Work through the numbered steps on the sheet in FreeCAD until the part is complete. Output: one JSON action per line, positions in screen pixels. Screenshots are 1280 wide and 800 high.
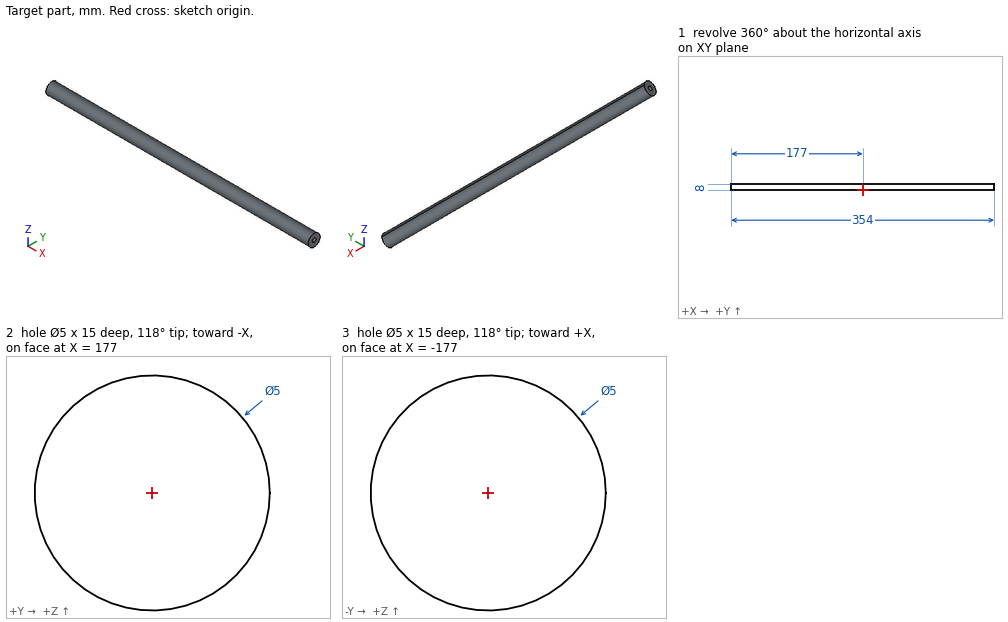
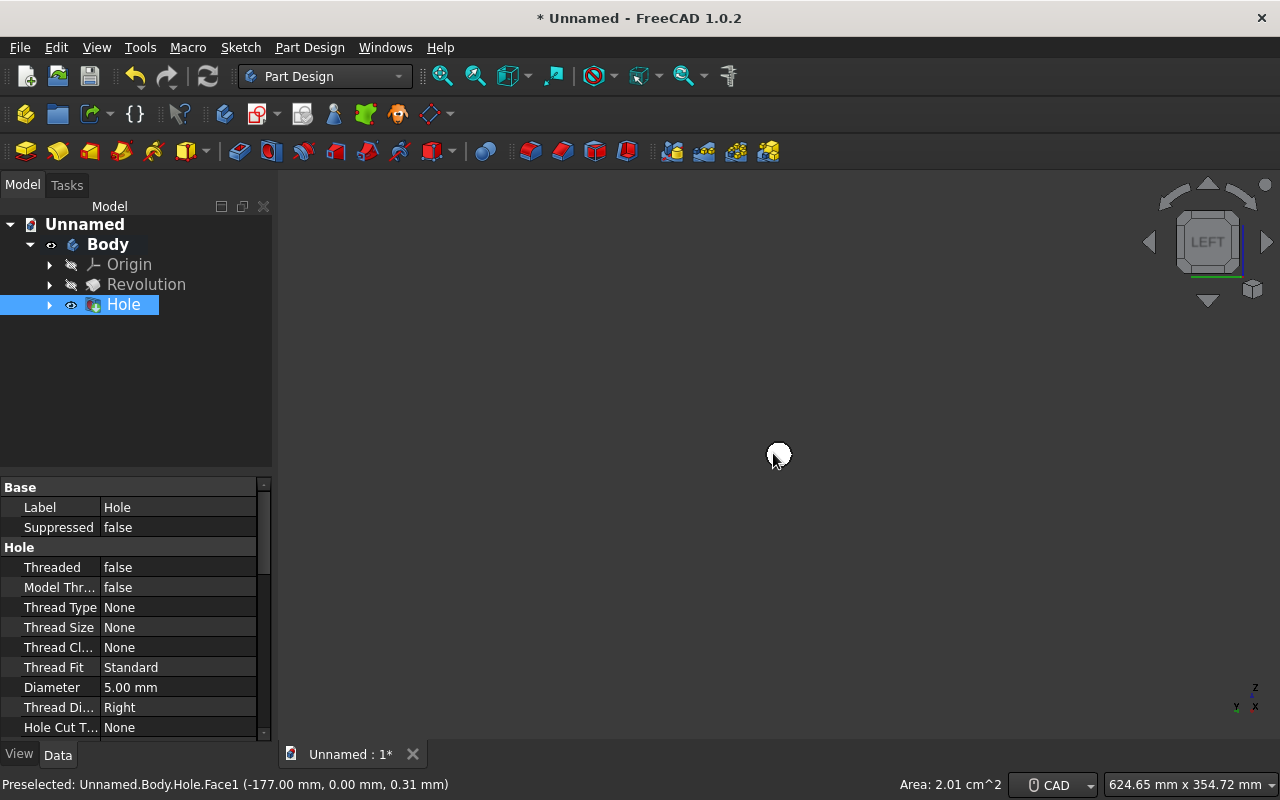
{"action": "left_click", "coordinate": [258, 114]}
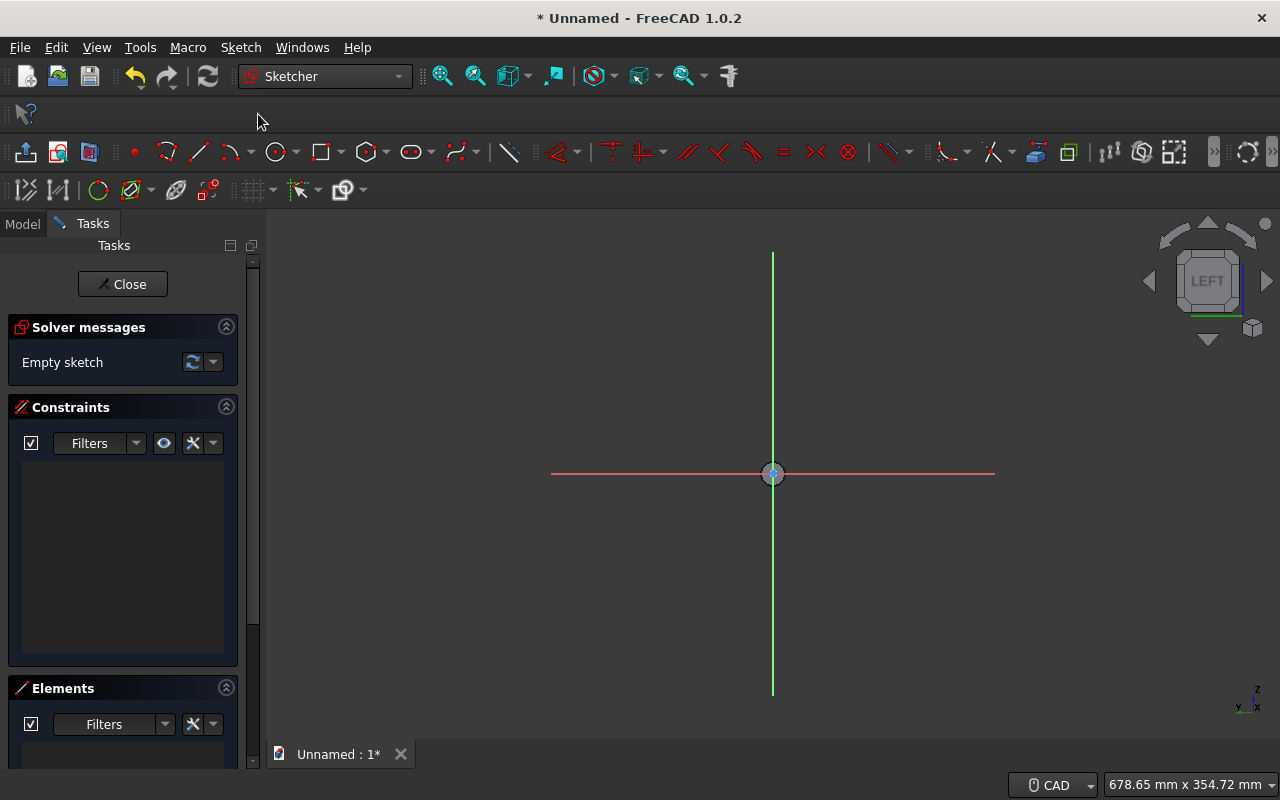
{"action": "scroll", "coordinate": [777, 474], "scroll_direction": "up", "scroll_amount": 15}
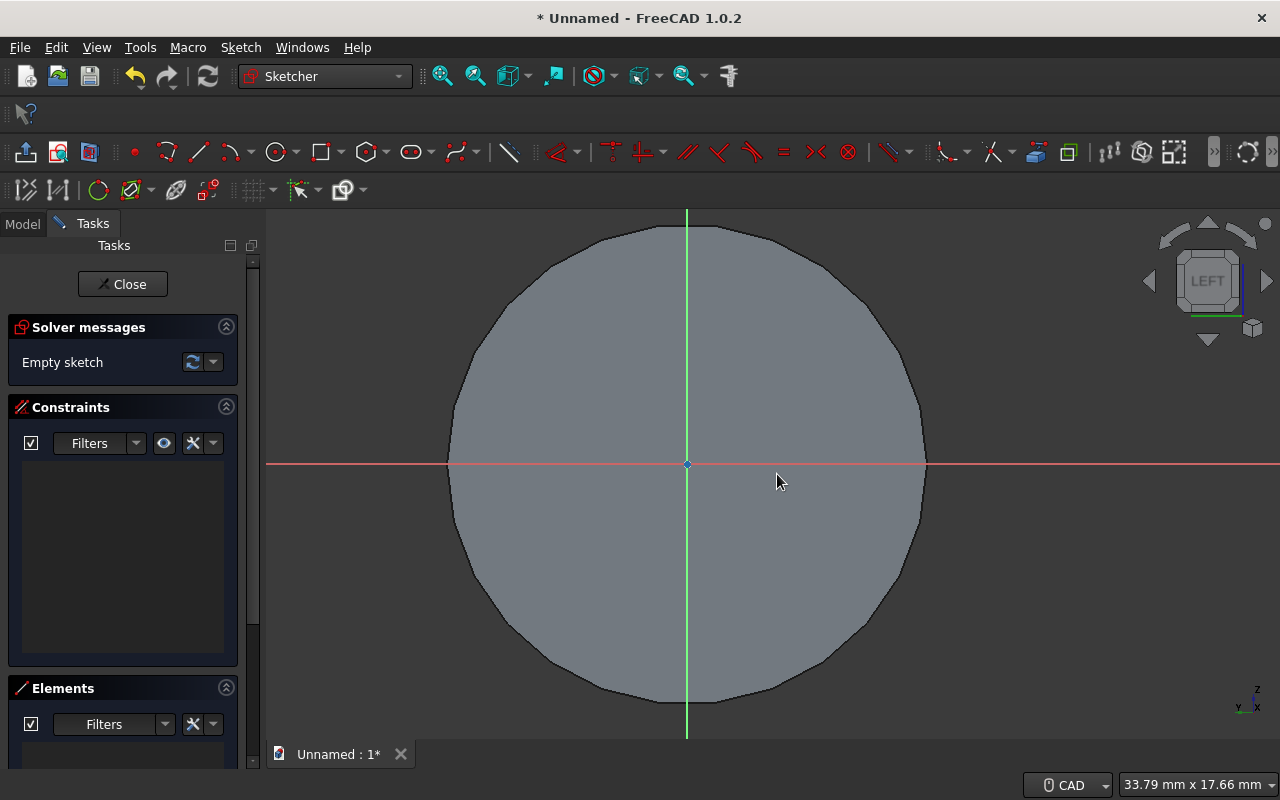
{"action": "scroll", "coordinate": [673, 457], "scroll_direction": "up", "scroll_amount": 4}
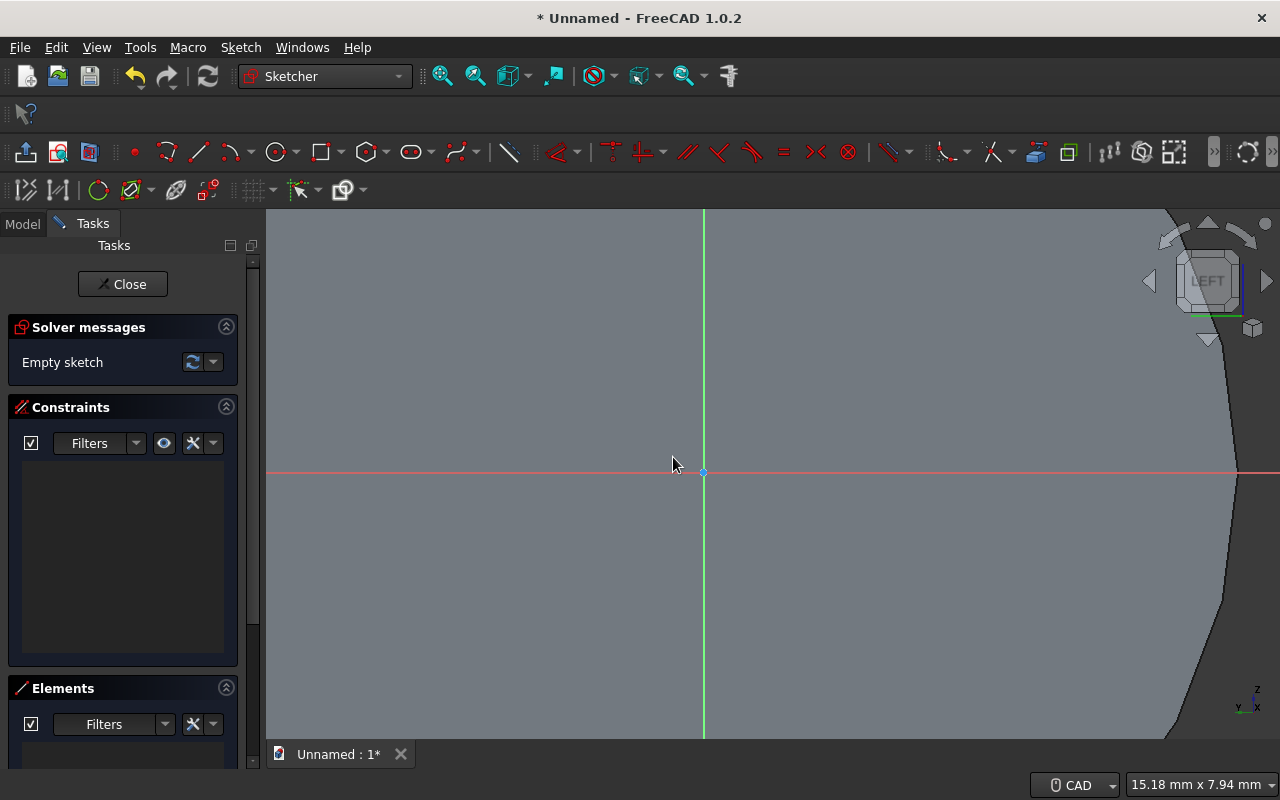
{"action": "left_click", "coordinate": [276, 152]}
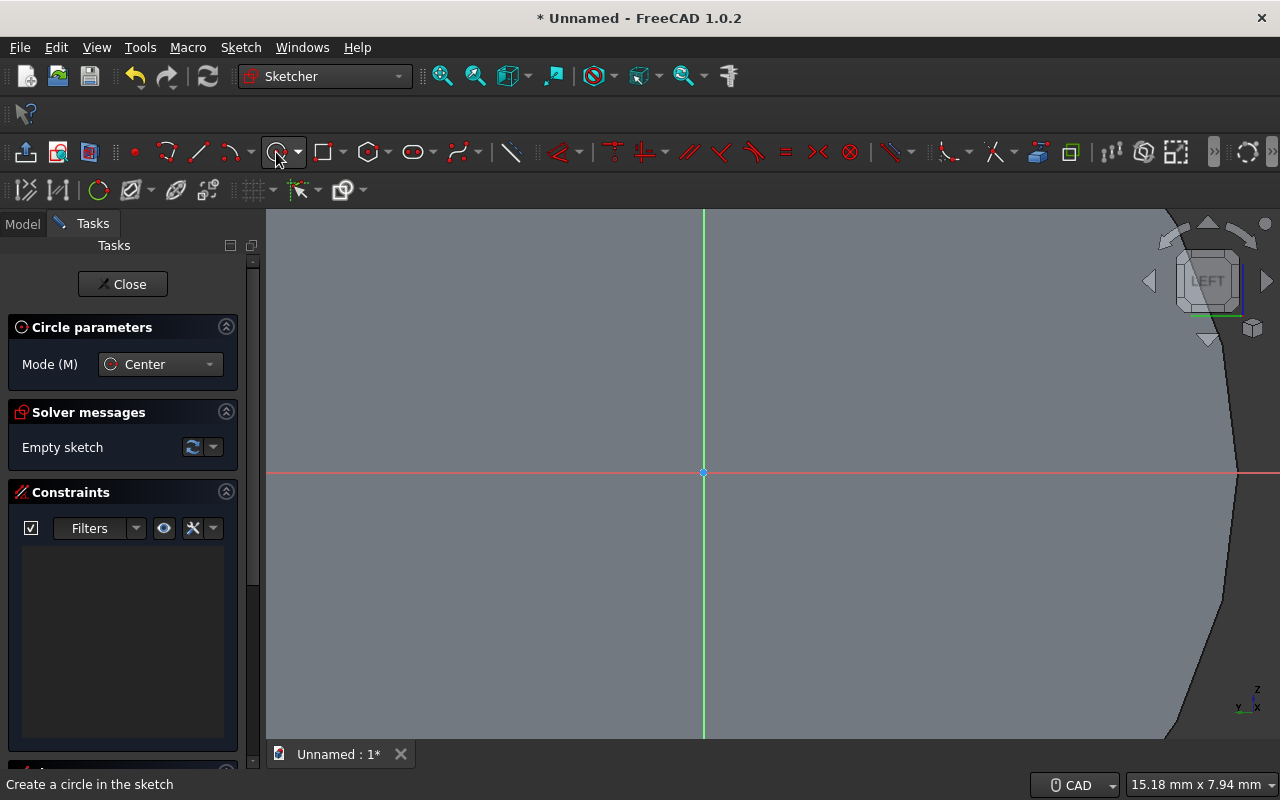
{"action": "left_click", "coordinate": [704, 473]}
{"action": "left_click", "coordinate": [822, 355]}
{"action": "key", "text": "Escape"}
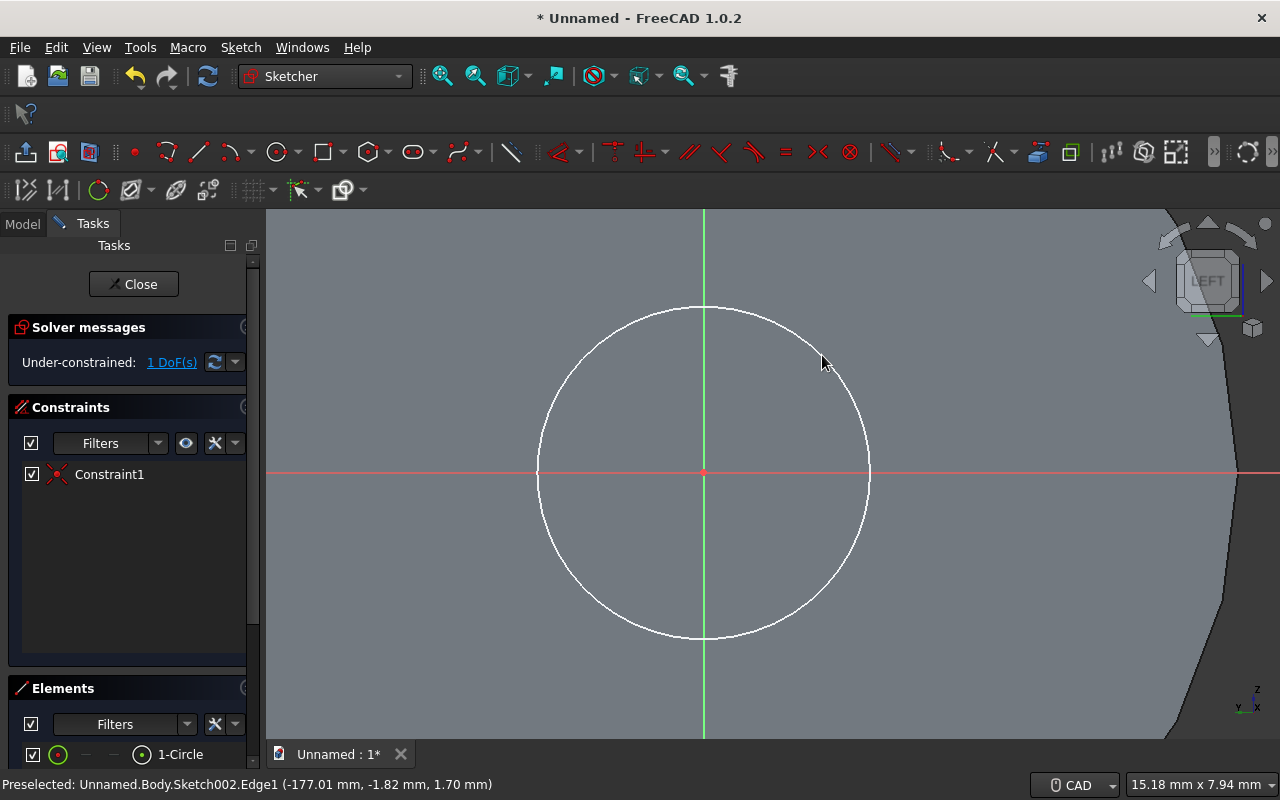
{"action": "left_click", "coordinate": [558, 152]}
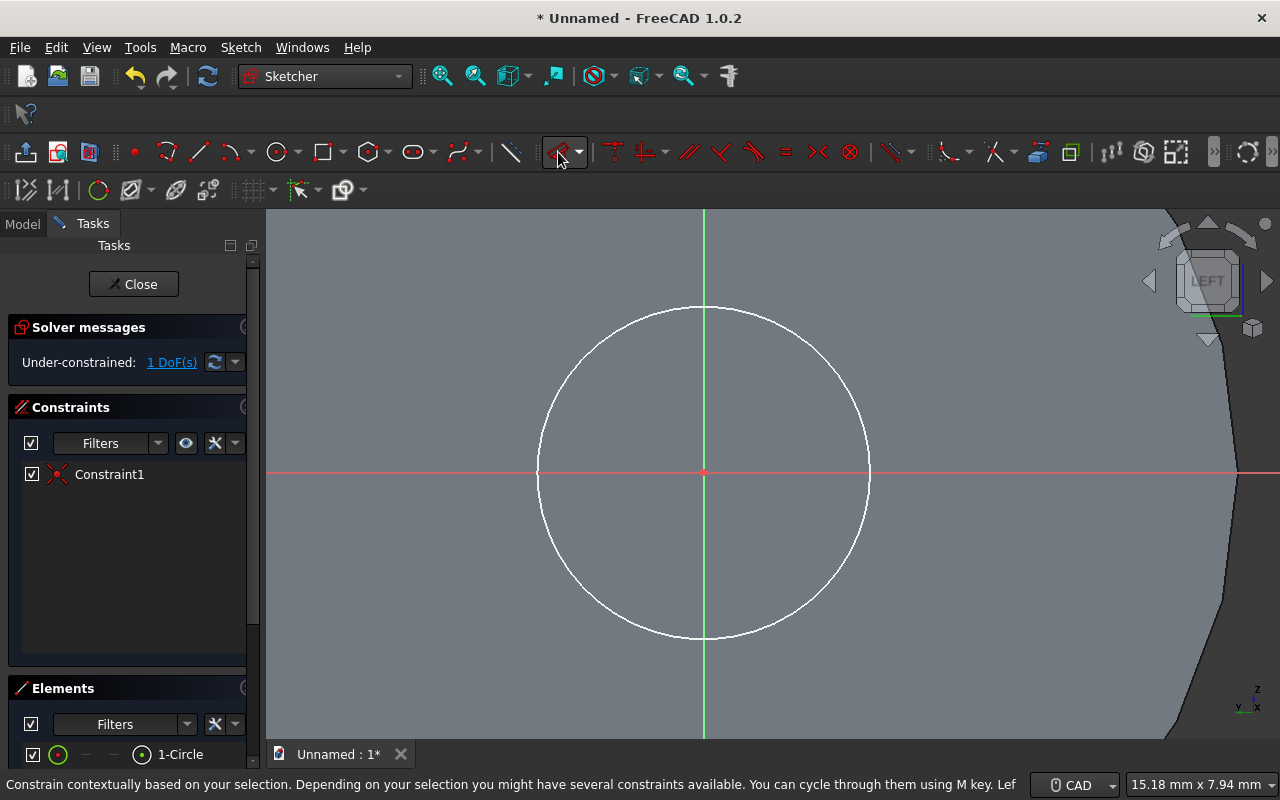
{"action": "left_click", "coordinate": [821, 355]}
{"action": "left_click", "coordinate": [844, 332]}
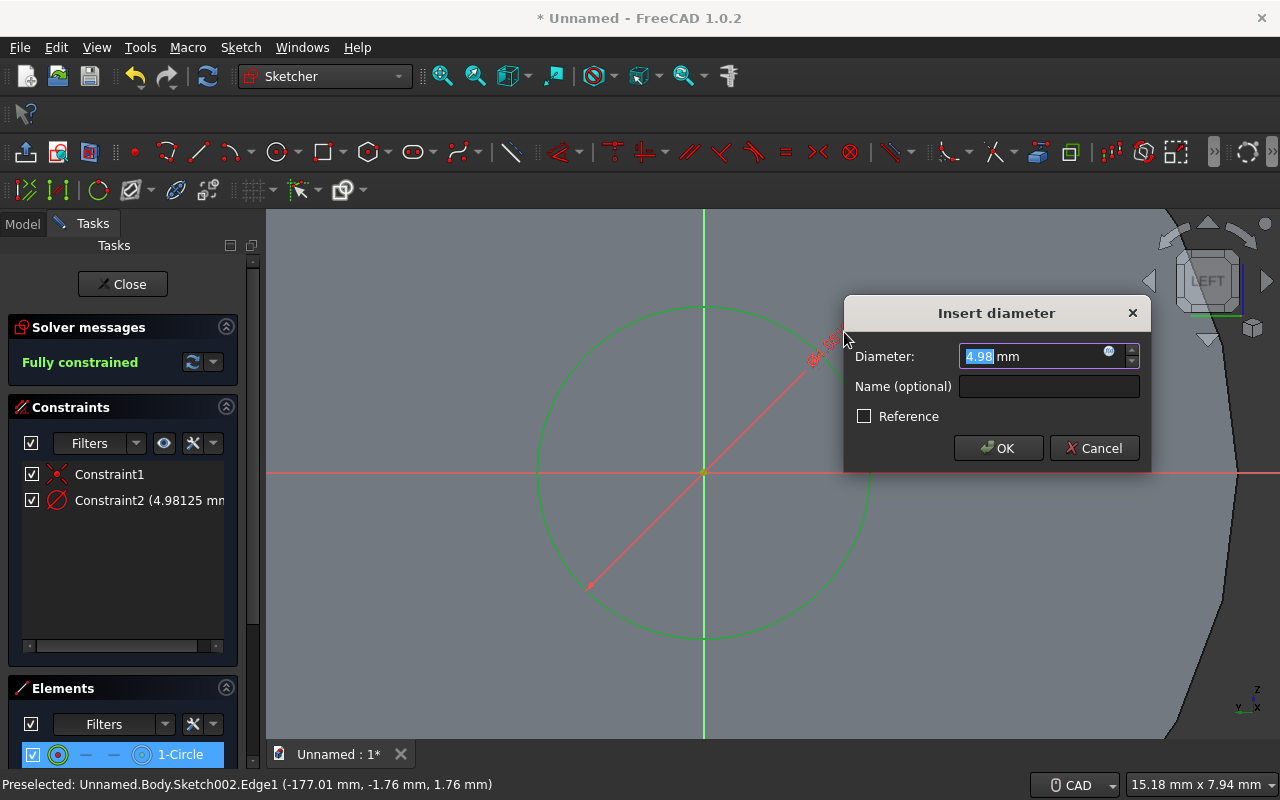
{"action": "type", "text": "5"}
{"action": "key", "text": "Return"}
{"action": "key", "text": "Escape"}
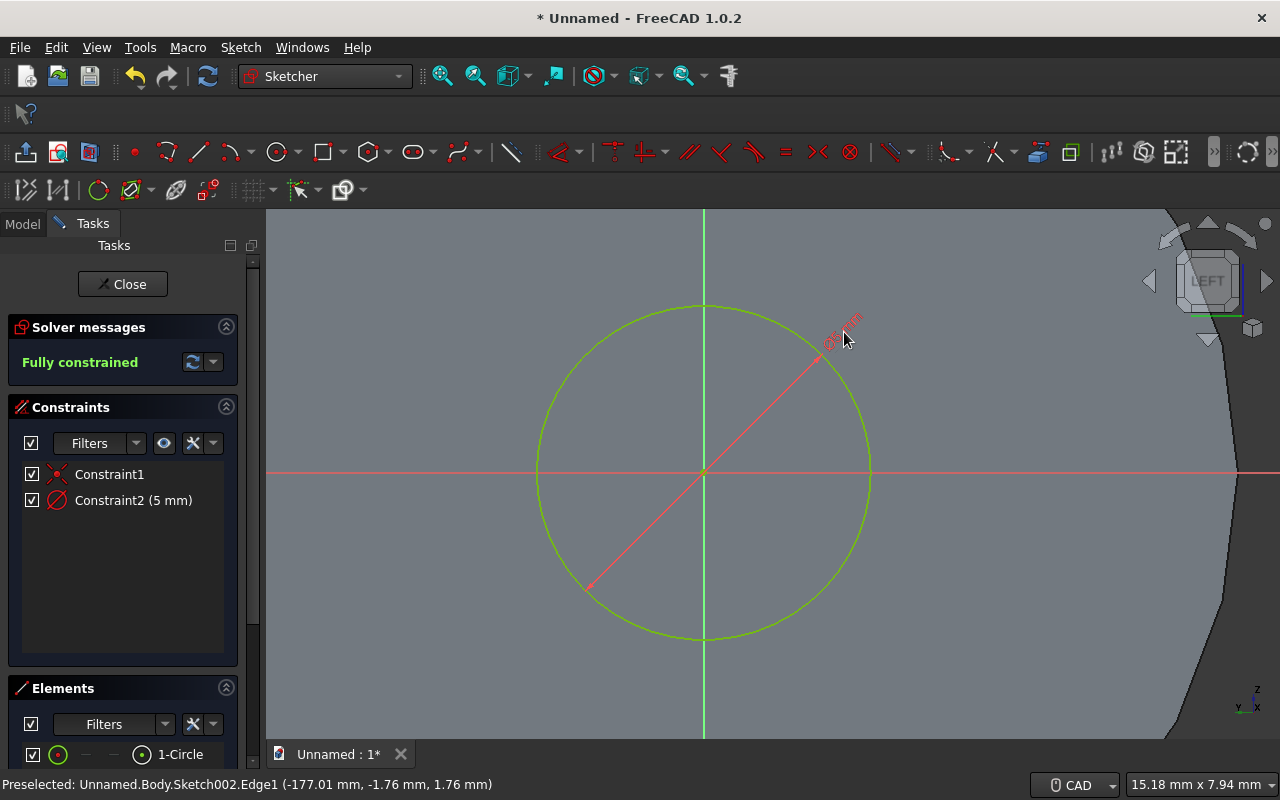
{"action": "left_click", "coordinate": [123, 284]}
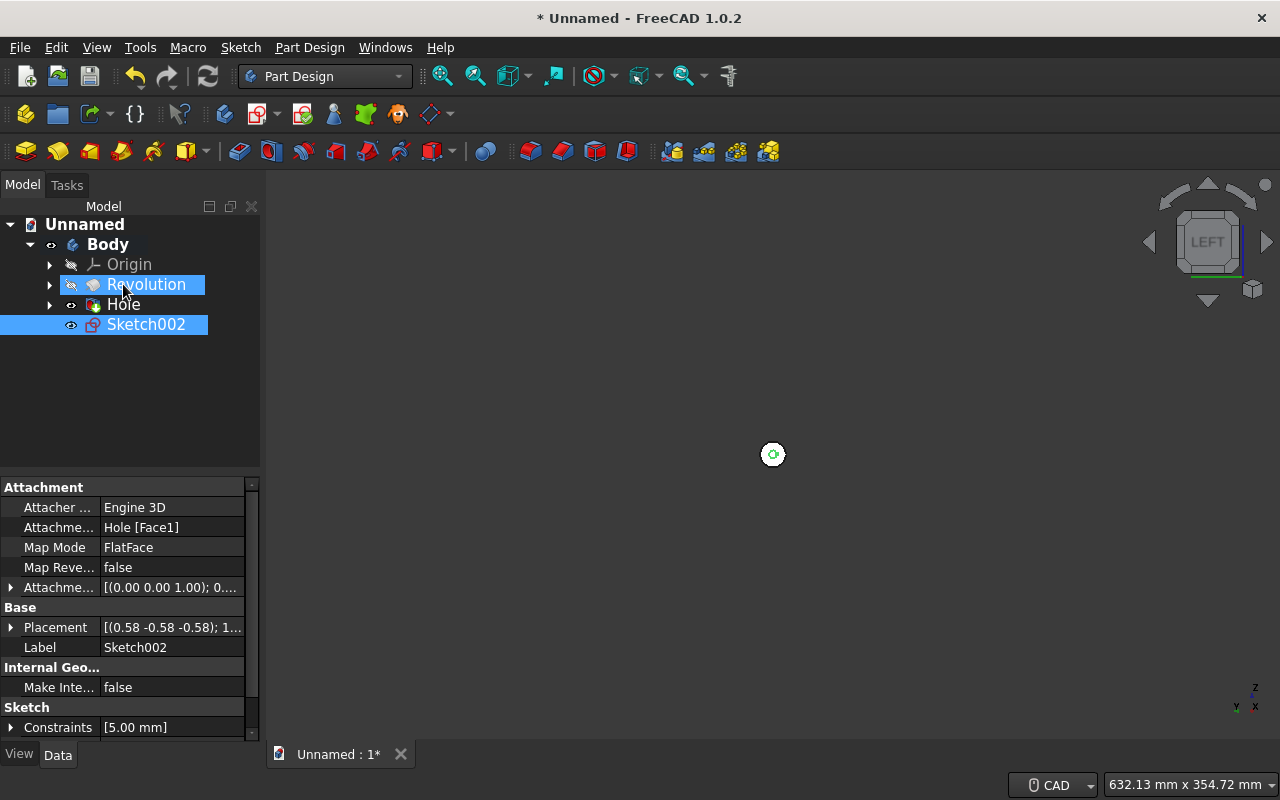
{"action": "left_click", "coordinate": [272, 152]}